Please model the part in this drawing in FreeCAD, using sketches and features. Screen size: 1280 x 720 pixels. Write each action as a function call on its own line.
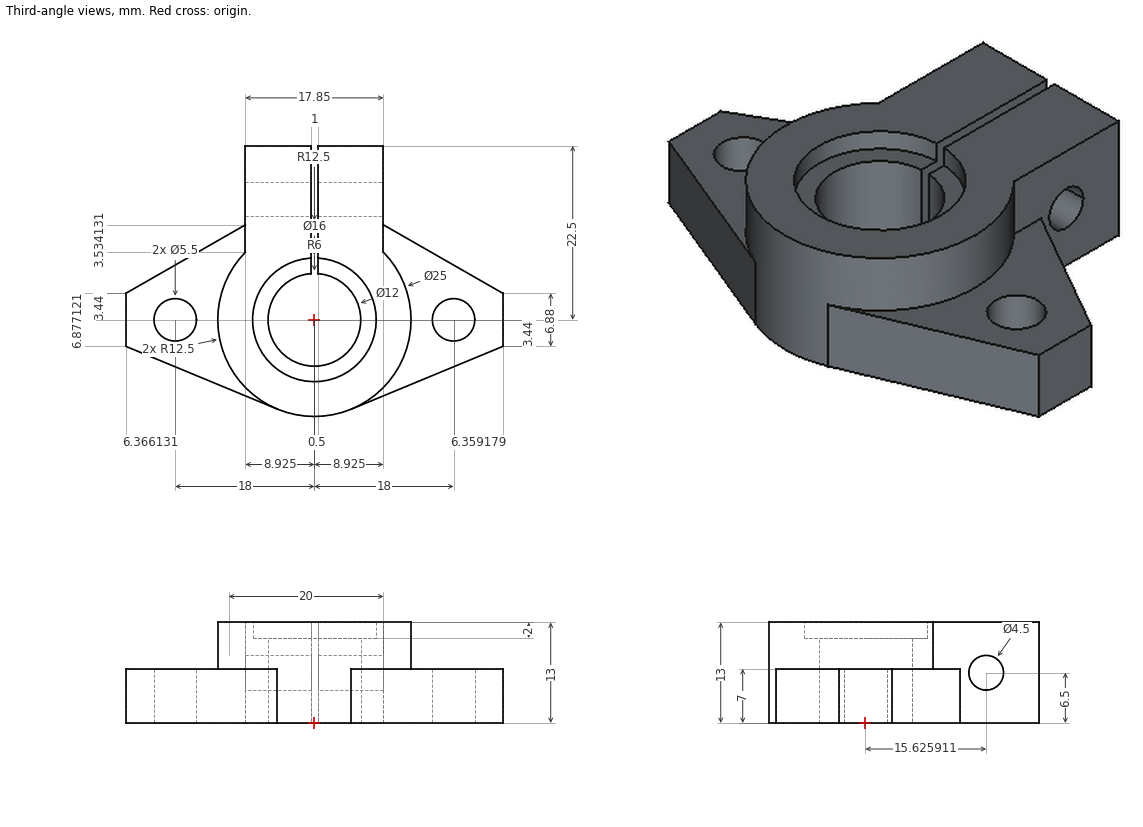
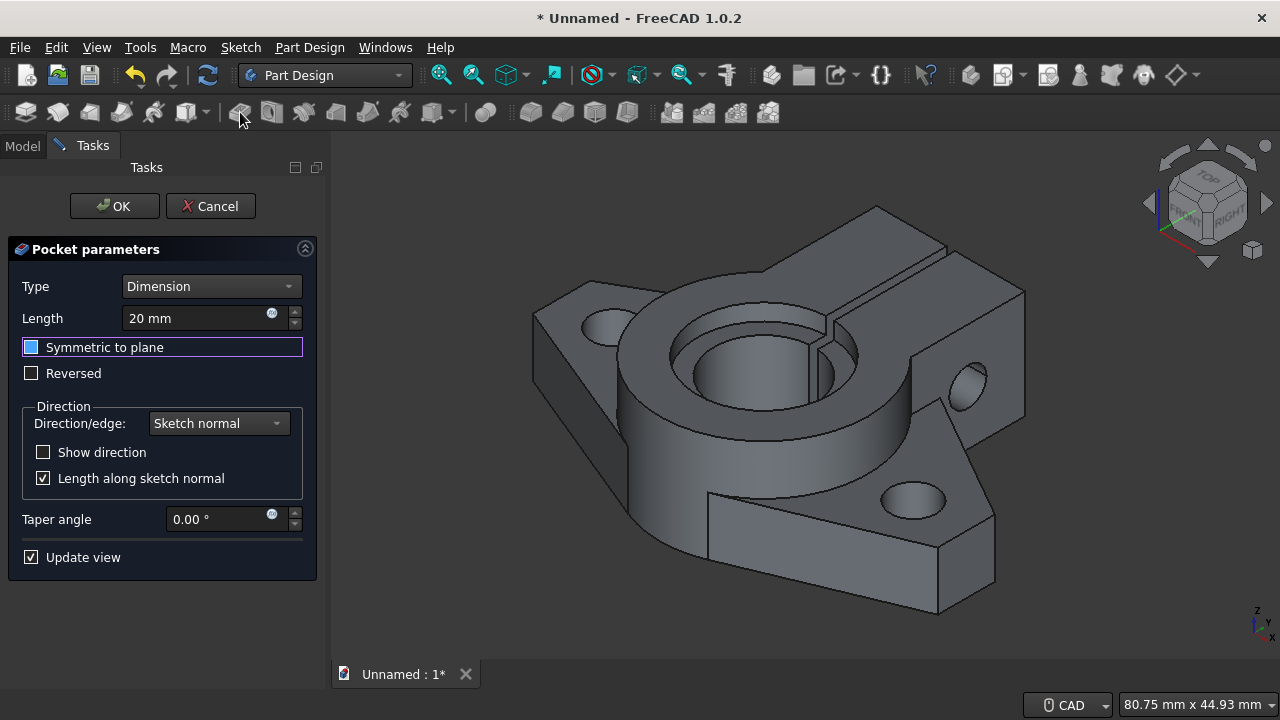
click(115, 206)